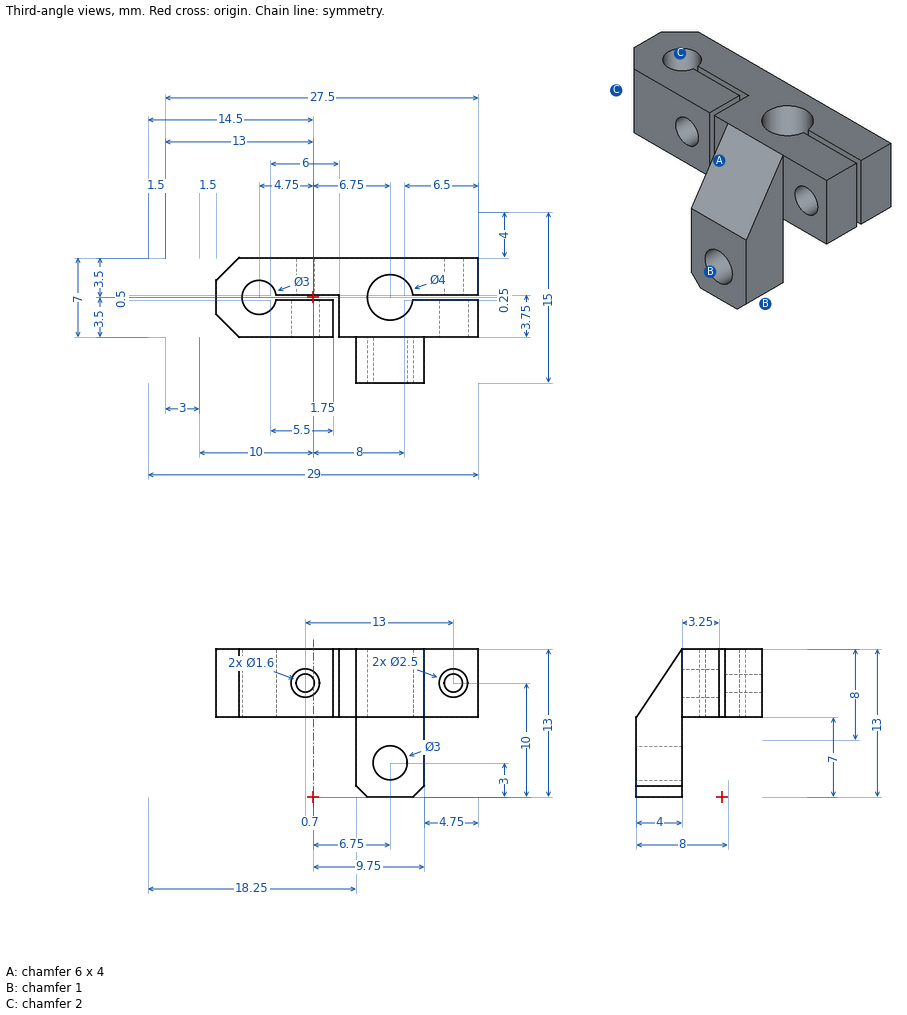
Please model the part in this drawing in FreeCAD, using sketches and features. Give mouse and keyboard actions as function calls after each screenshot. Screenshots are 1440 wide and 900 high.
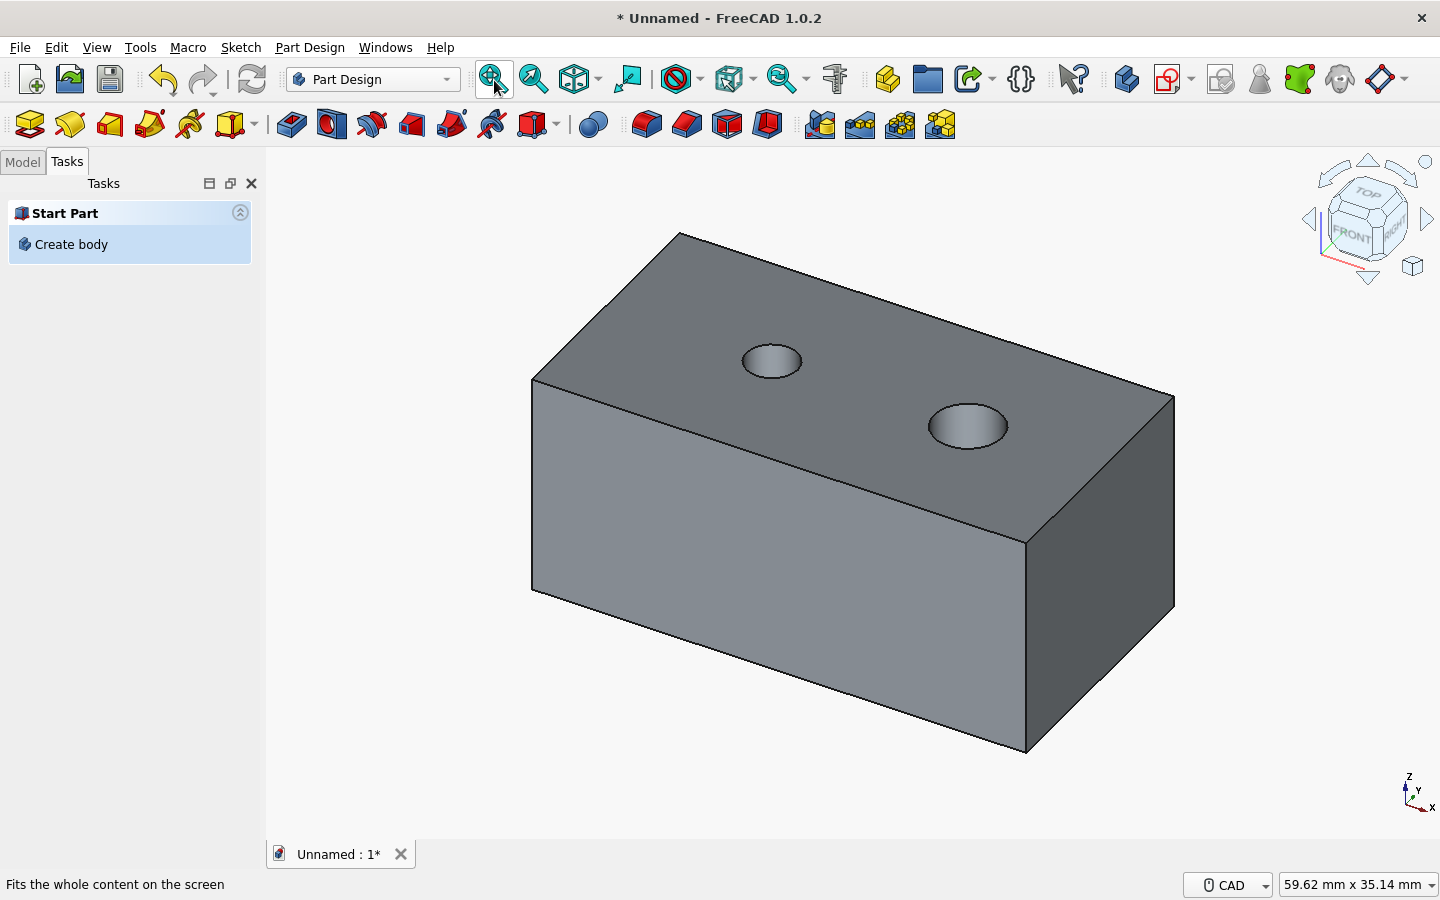
click(850, 589)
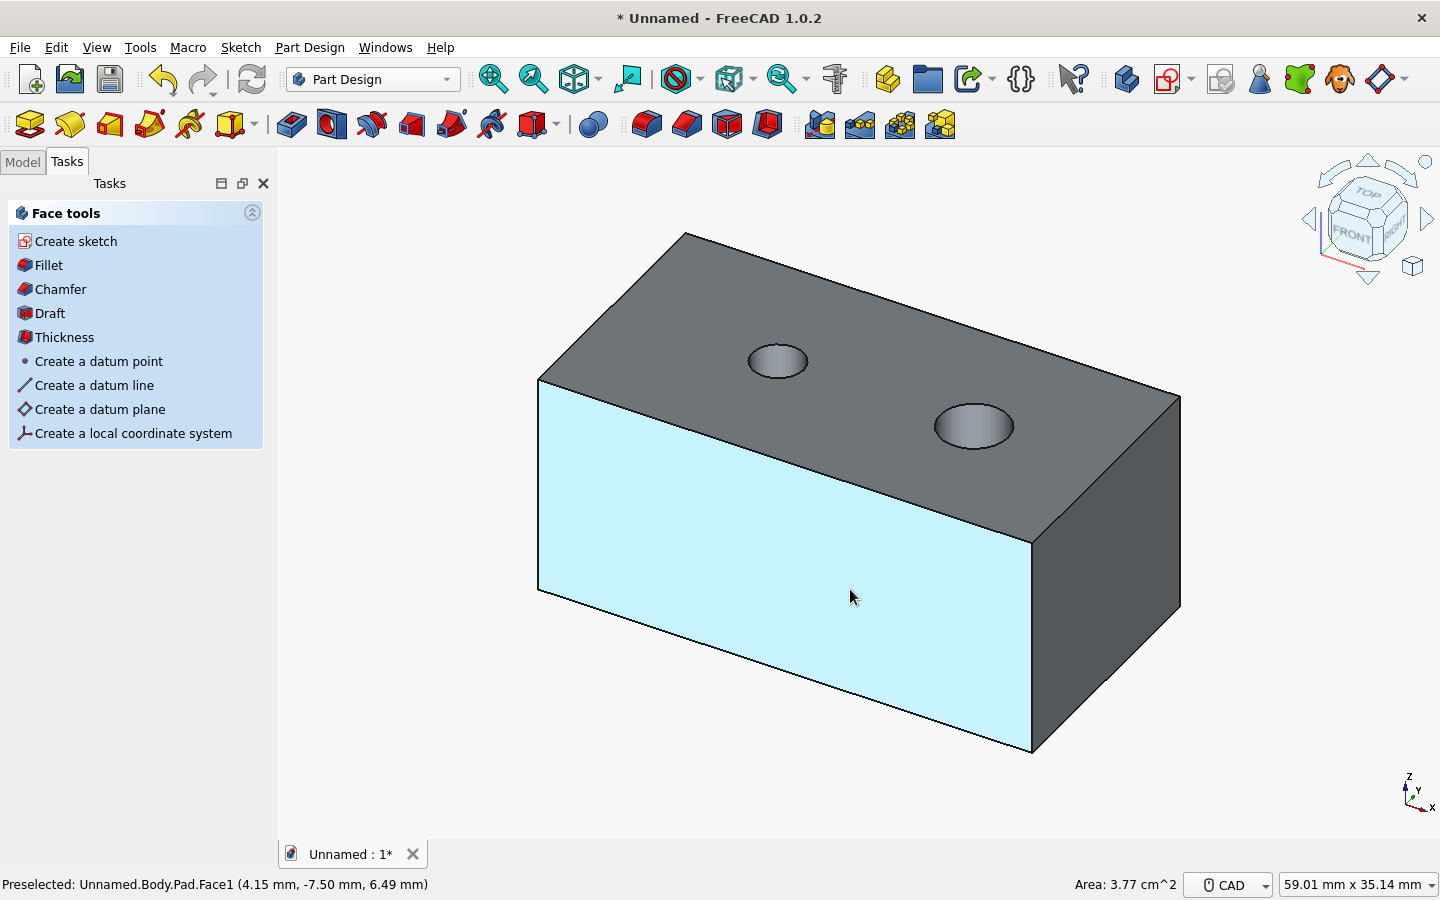
click(1168, 80)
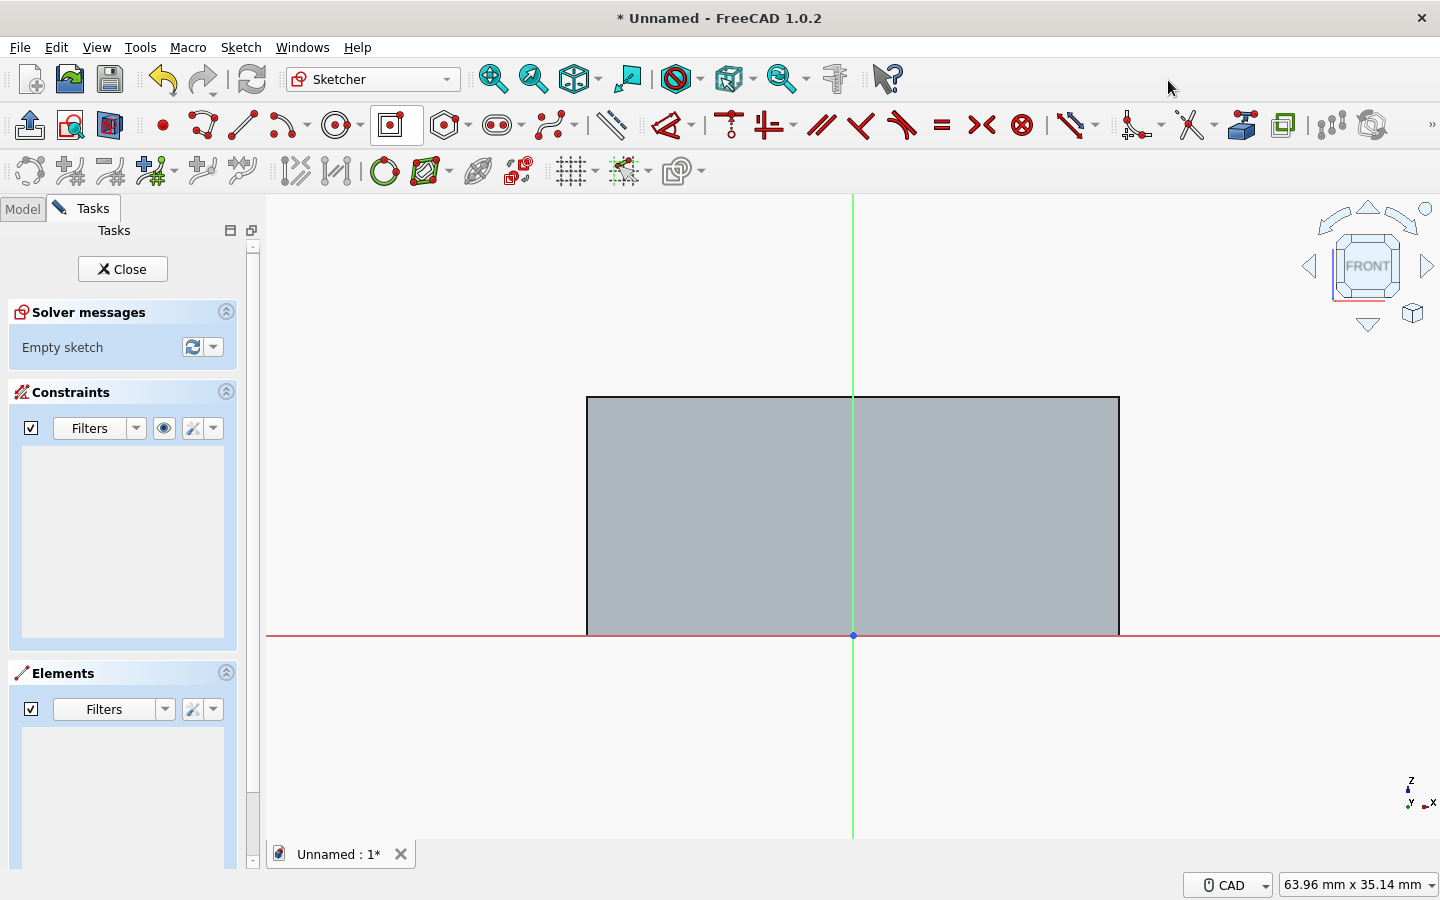
click(418, 126)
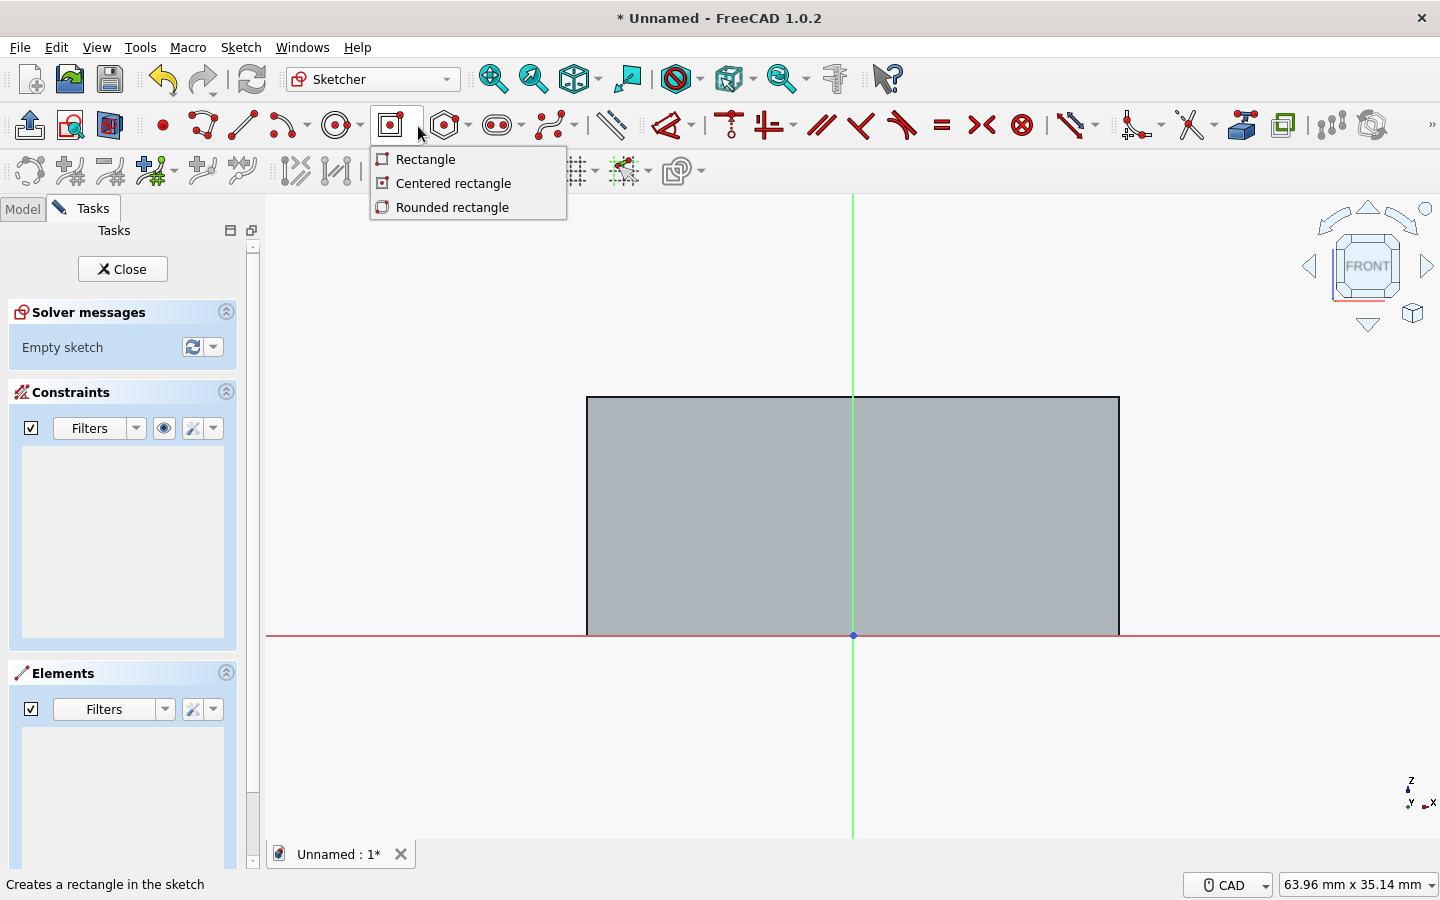
click(468, 159)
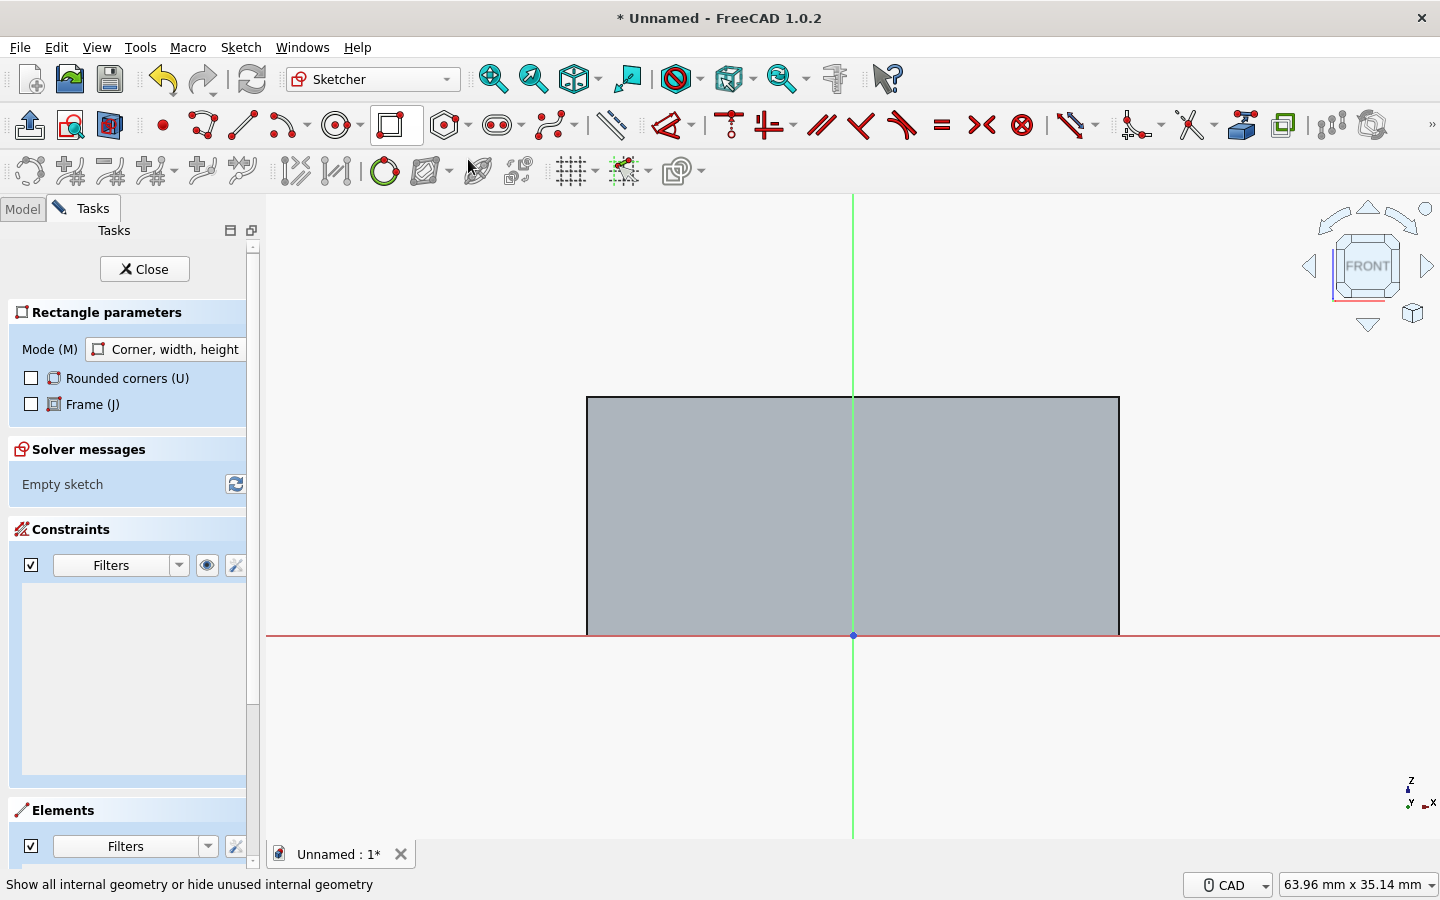
click(1032, 397)
click(1119, 636)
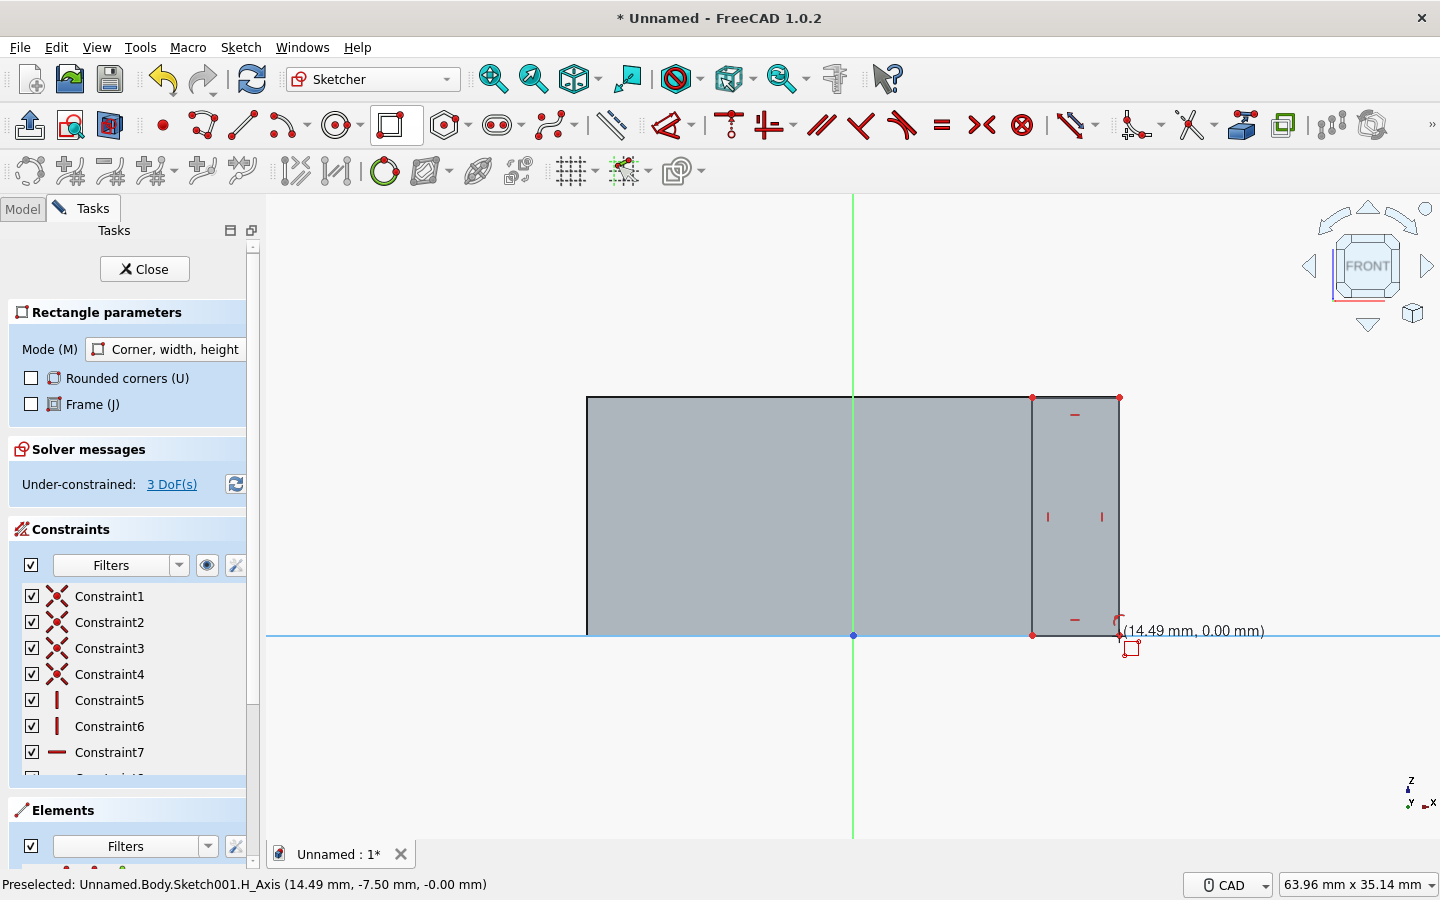
click(587, 397)
click(922, 636)
key(Escape)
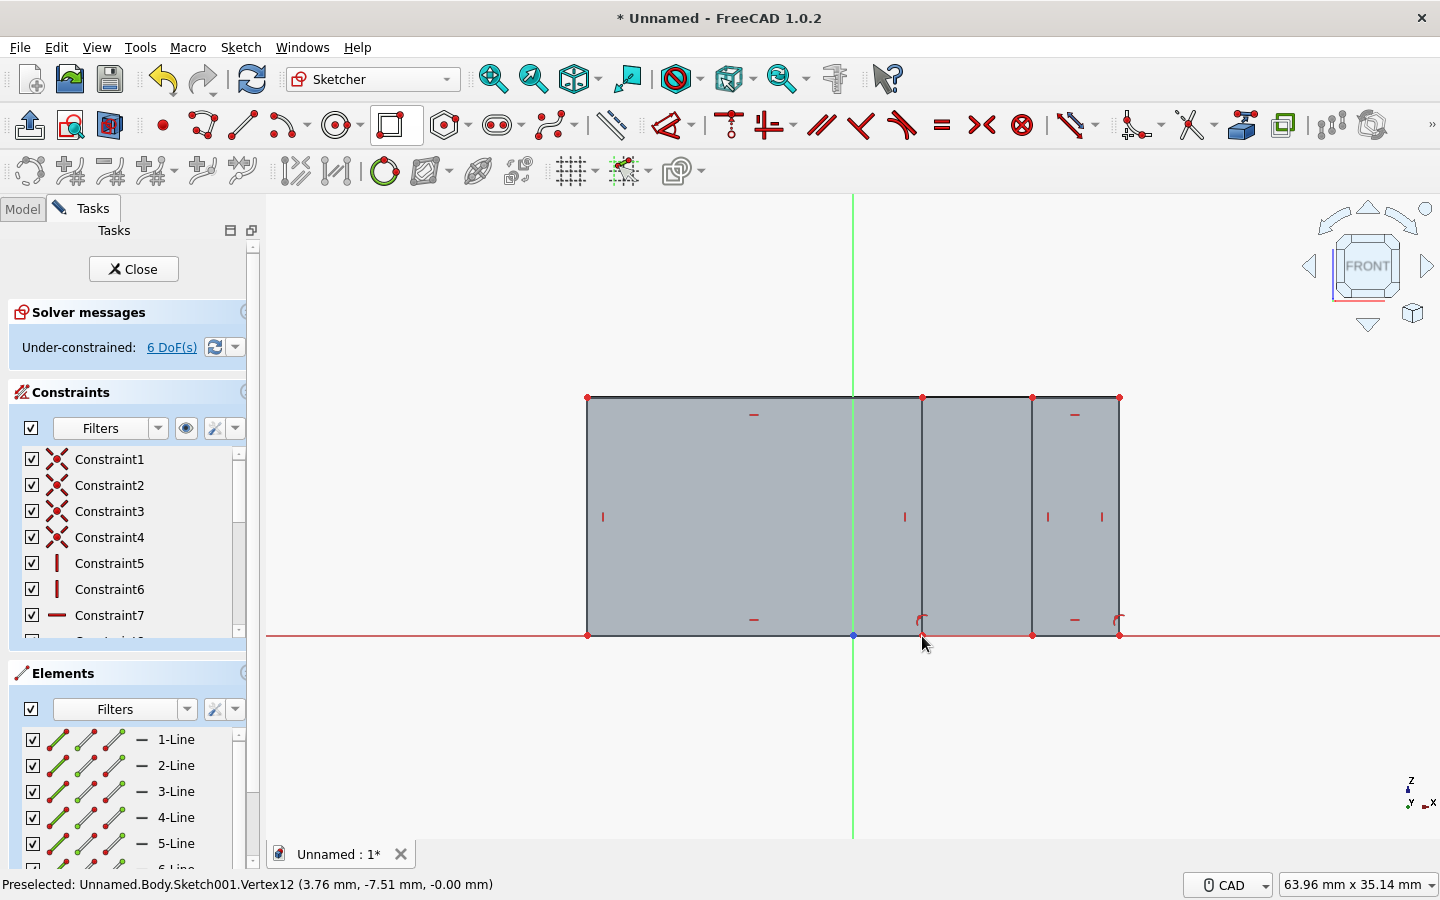
click(1119, 398)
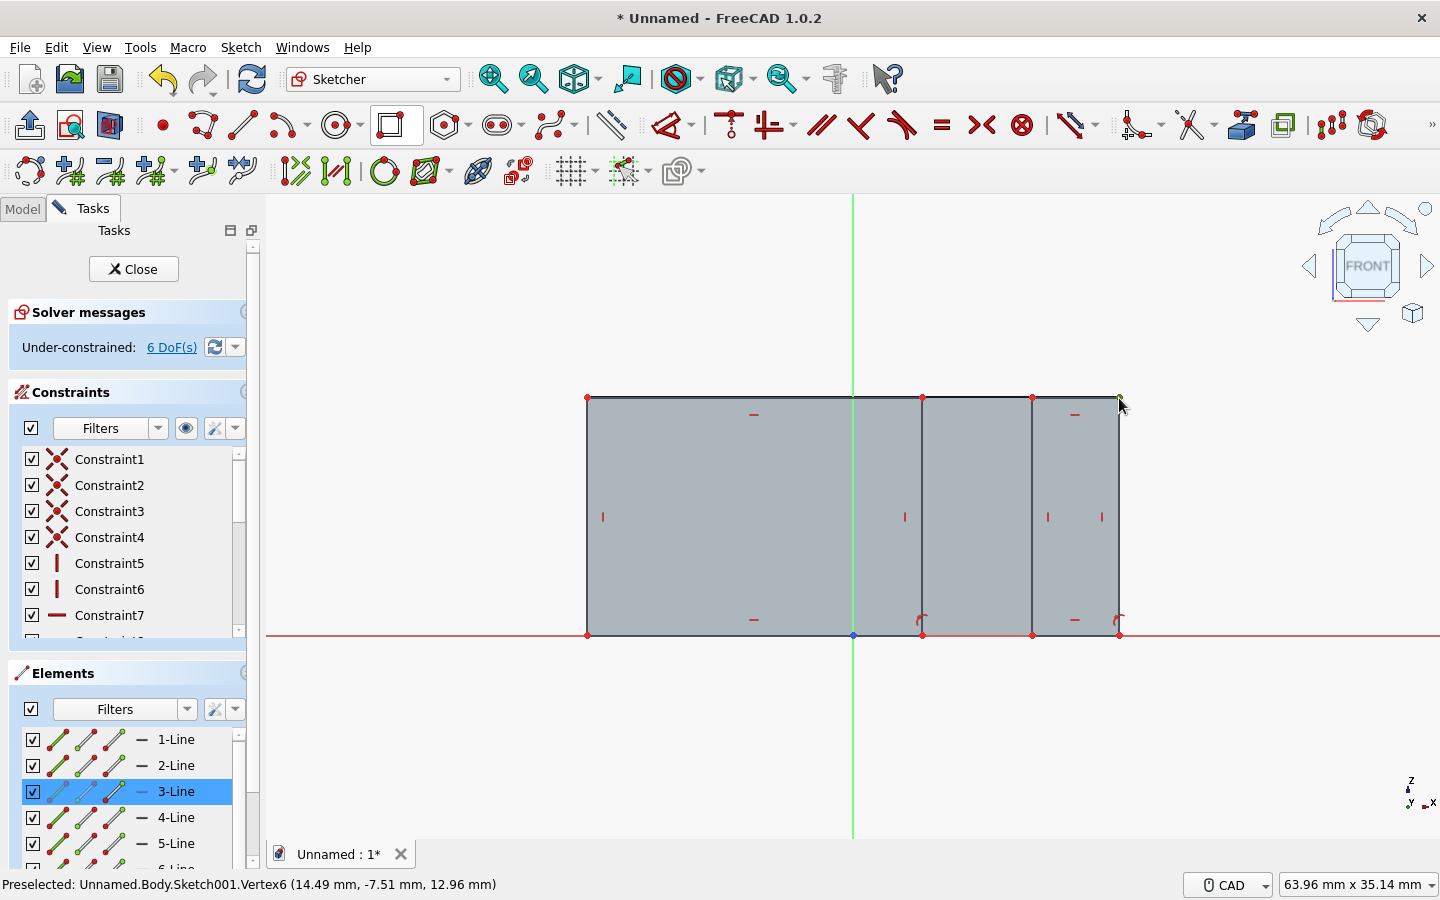
click(587, 398)